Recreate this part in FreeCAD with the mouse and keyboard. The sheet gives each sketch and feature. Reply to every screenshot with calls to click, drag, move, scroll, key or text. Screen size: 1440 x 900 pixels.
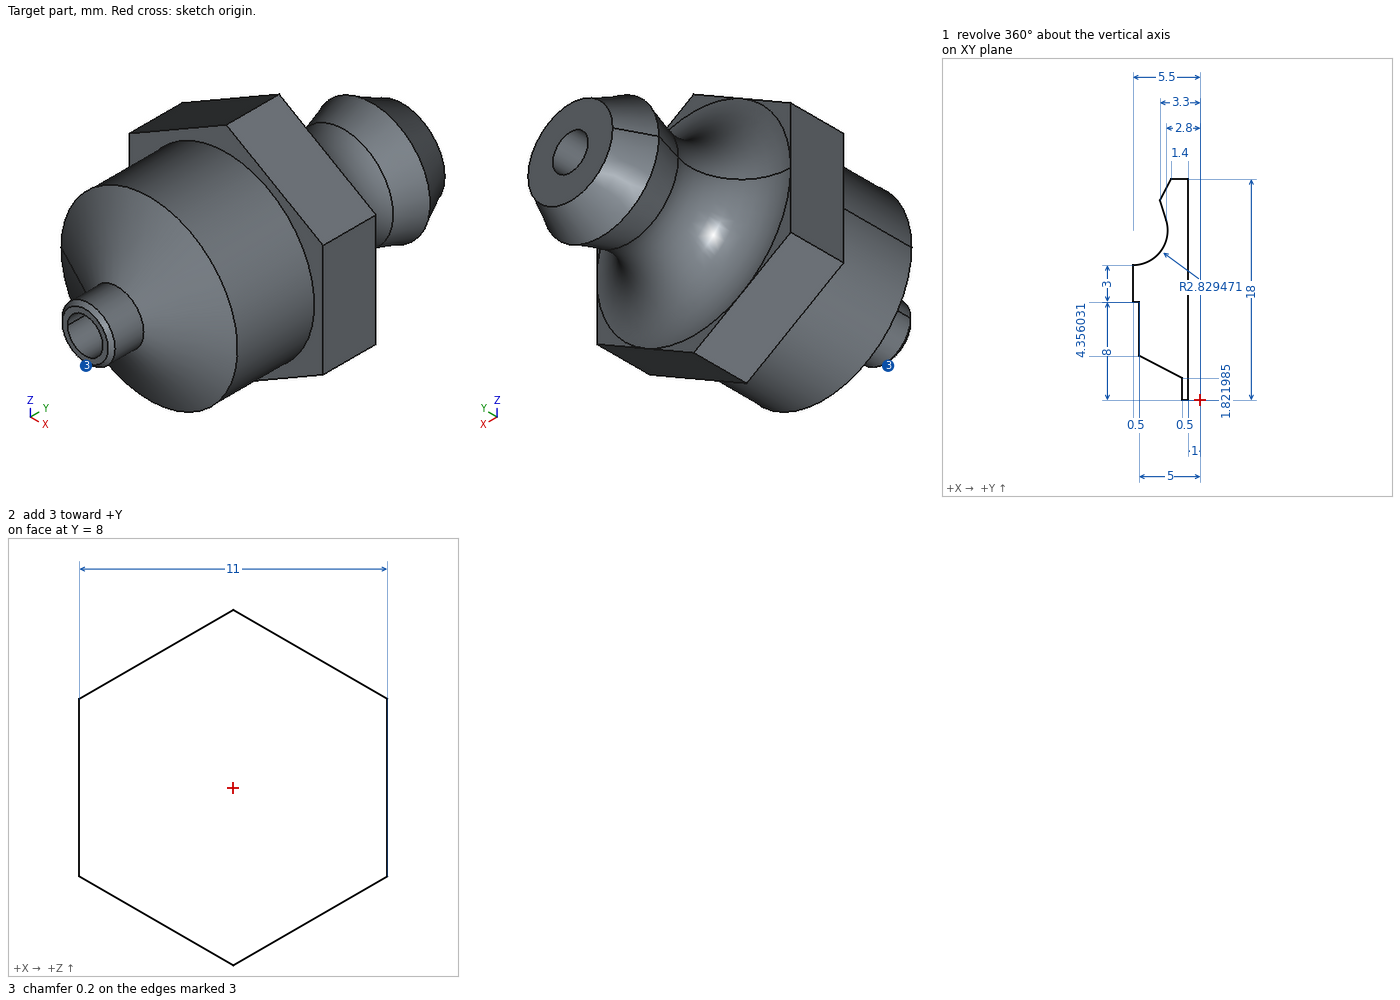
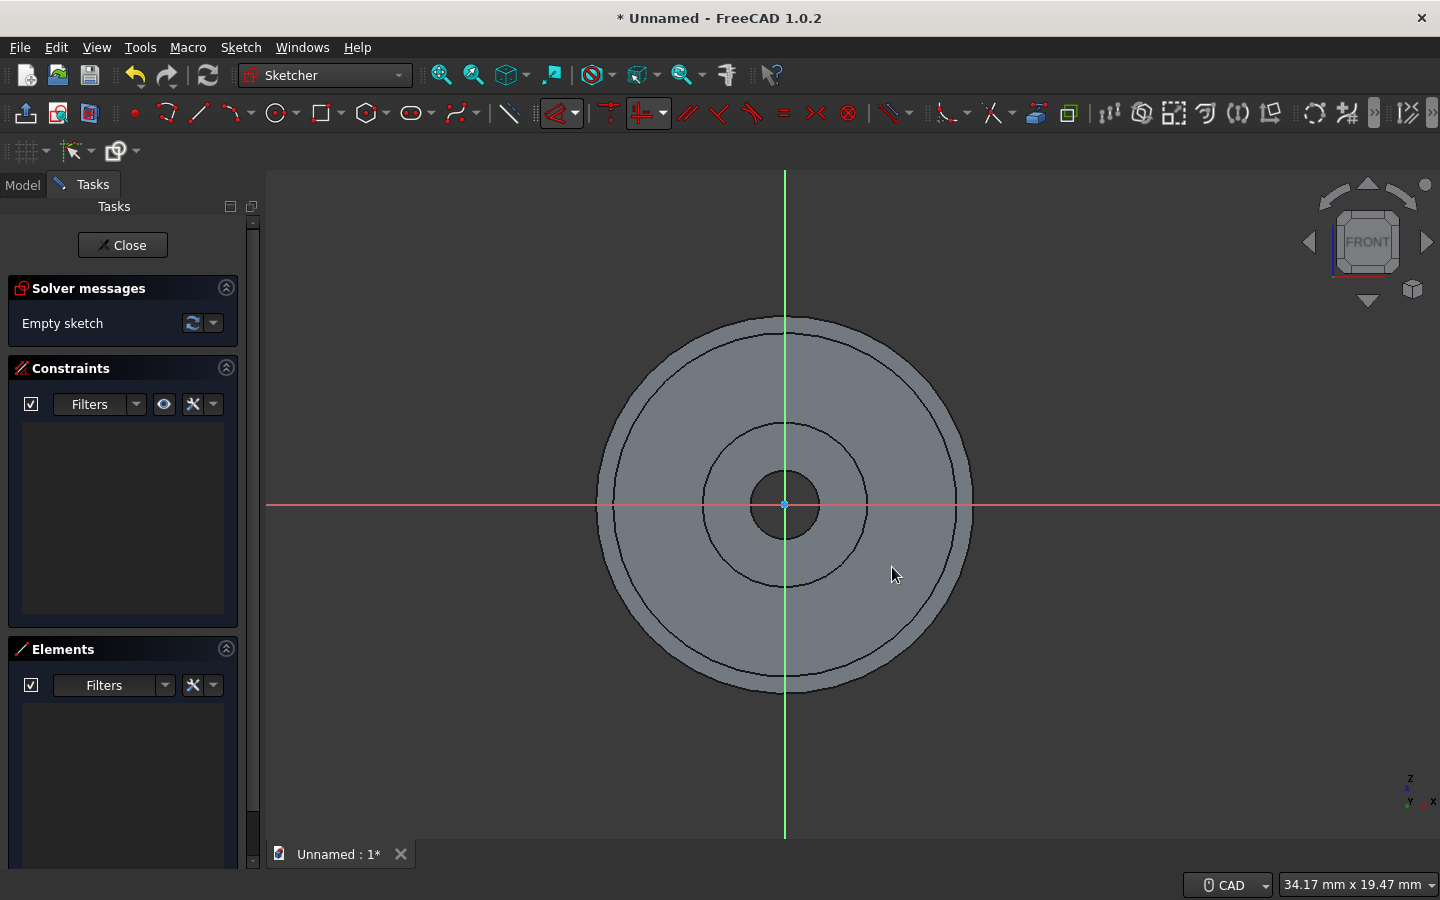
click(366, 114)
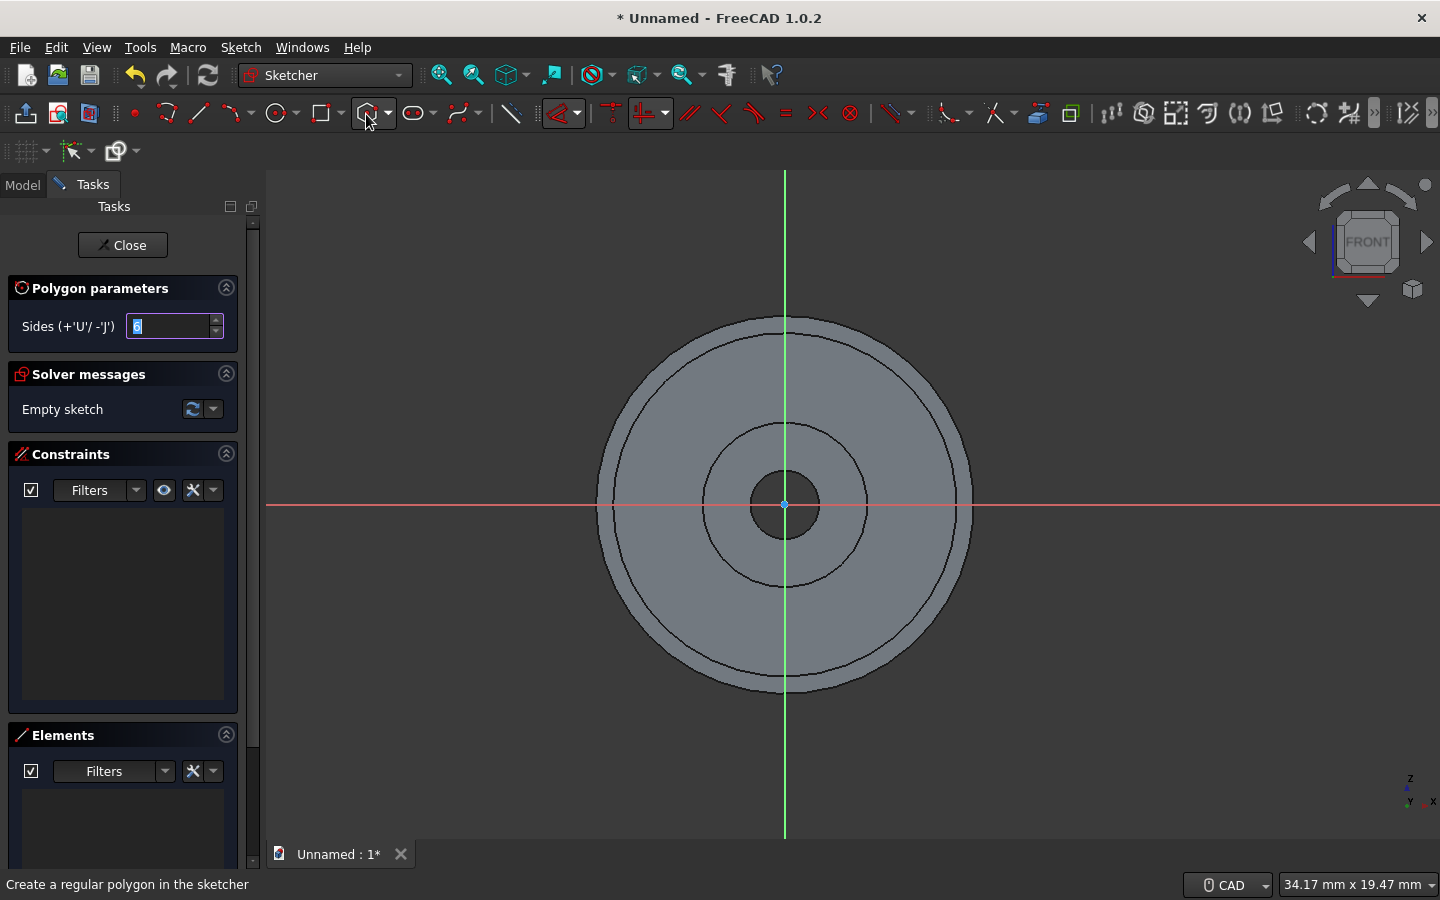
click(785, 505)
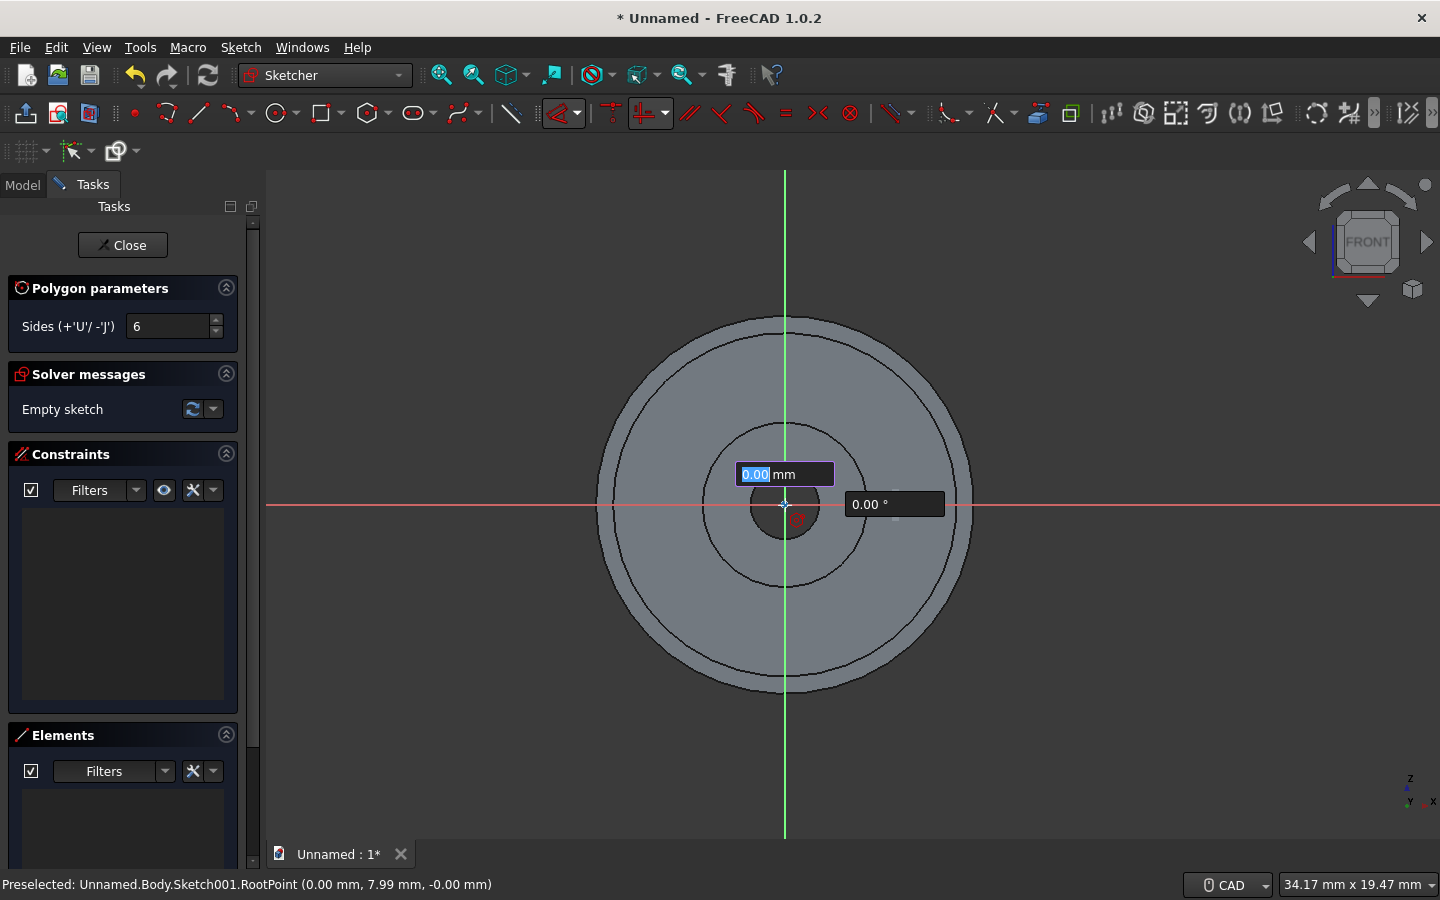
click(785, 723)
right_click(785, 723)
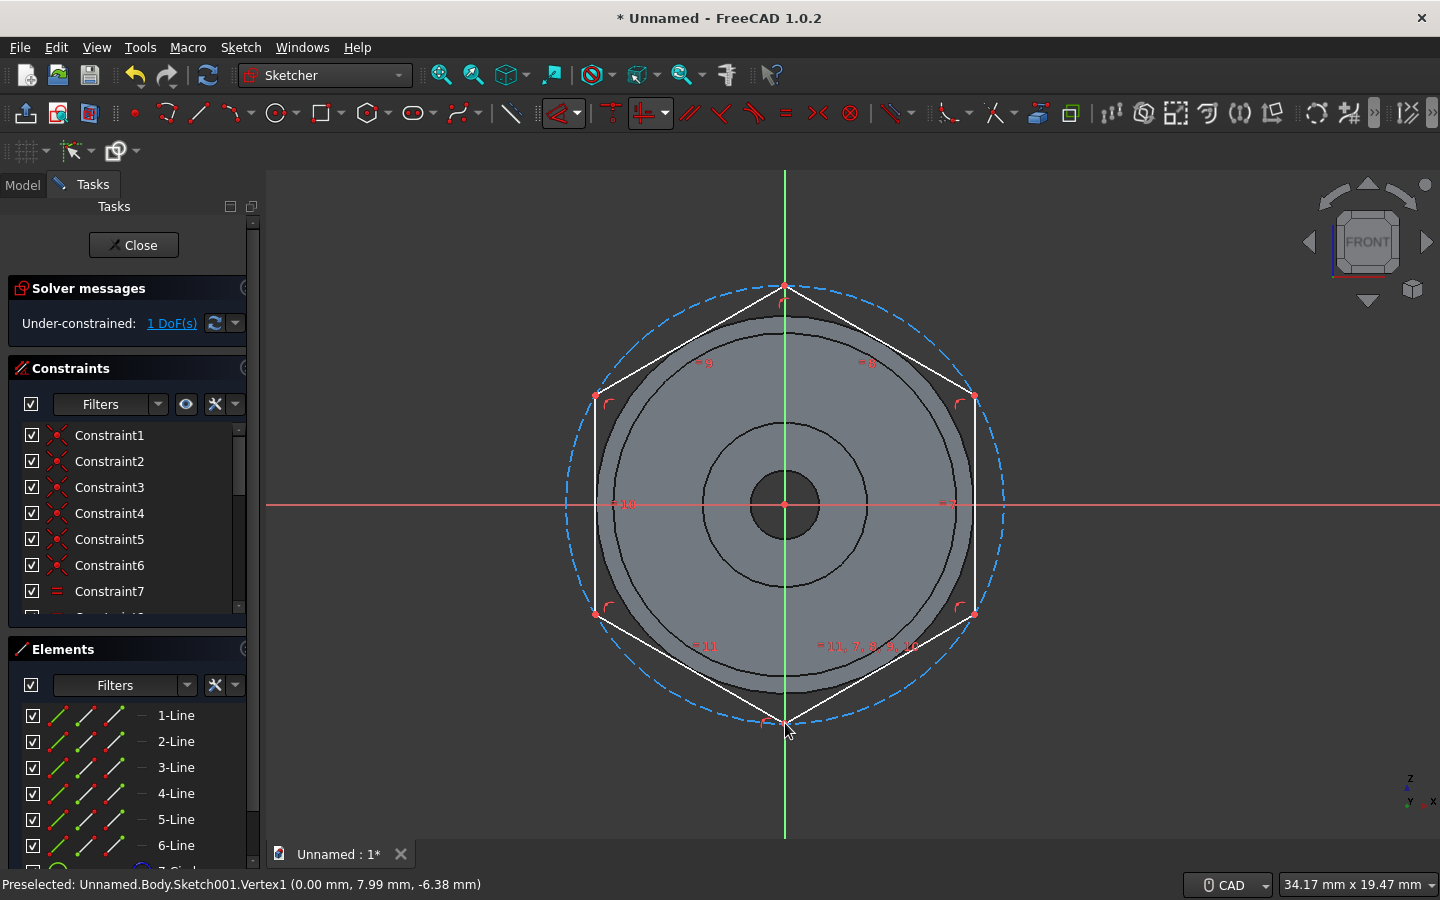
click(595, 395)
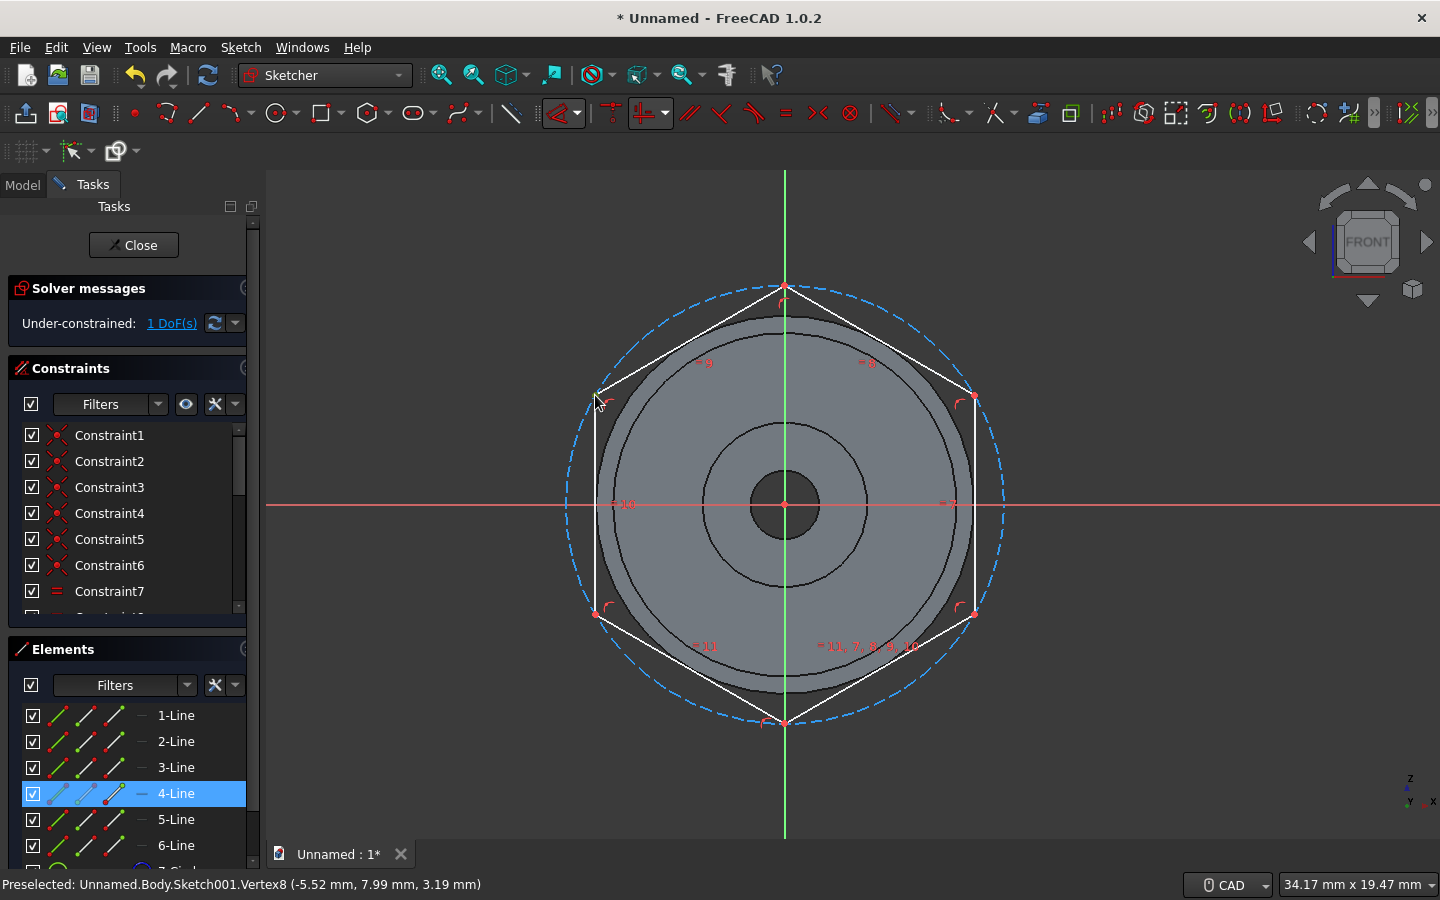
click(975, 614)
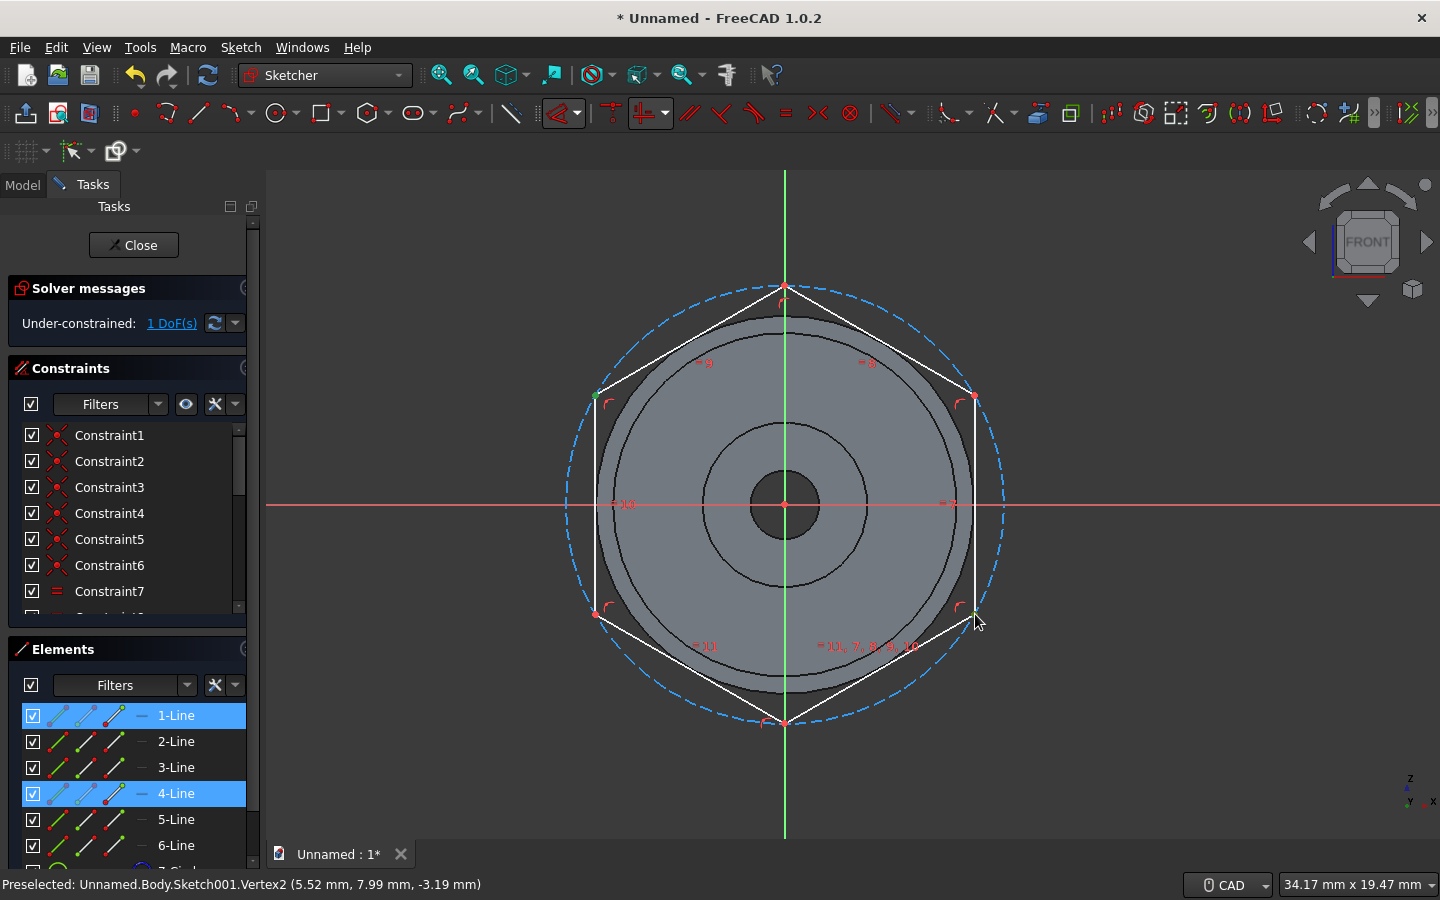
click(580, 114)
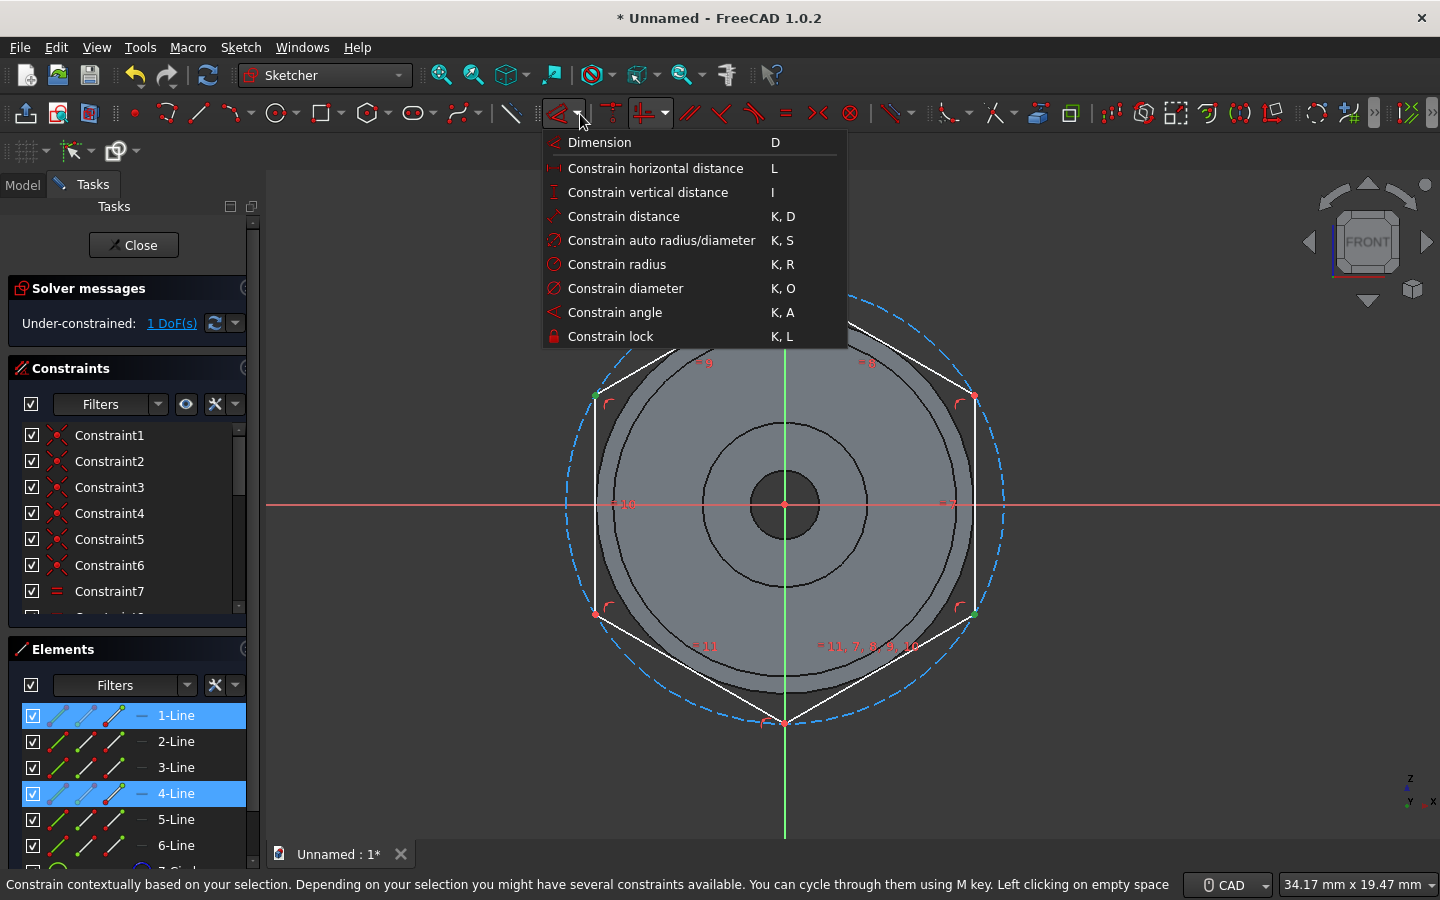
click(695, 168)